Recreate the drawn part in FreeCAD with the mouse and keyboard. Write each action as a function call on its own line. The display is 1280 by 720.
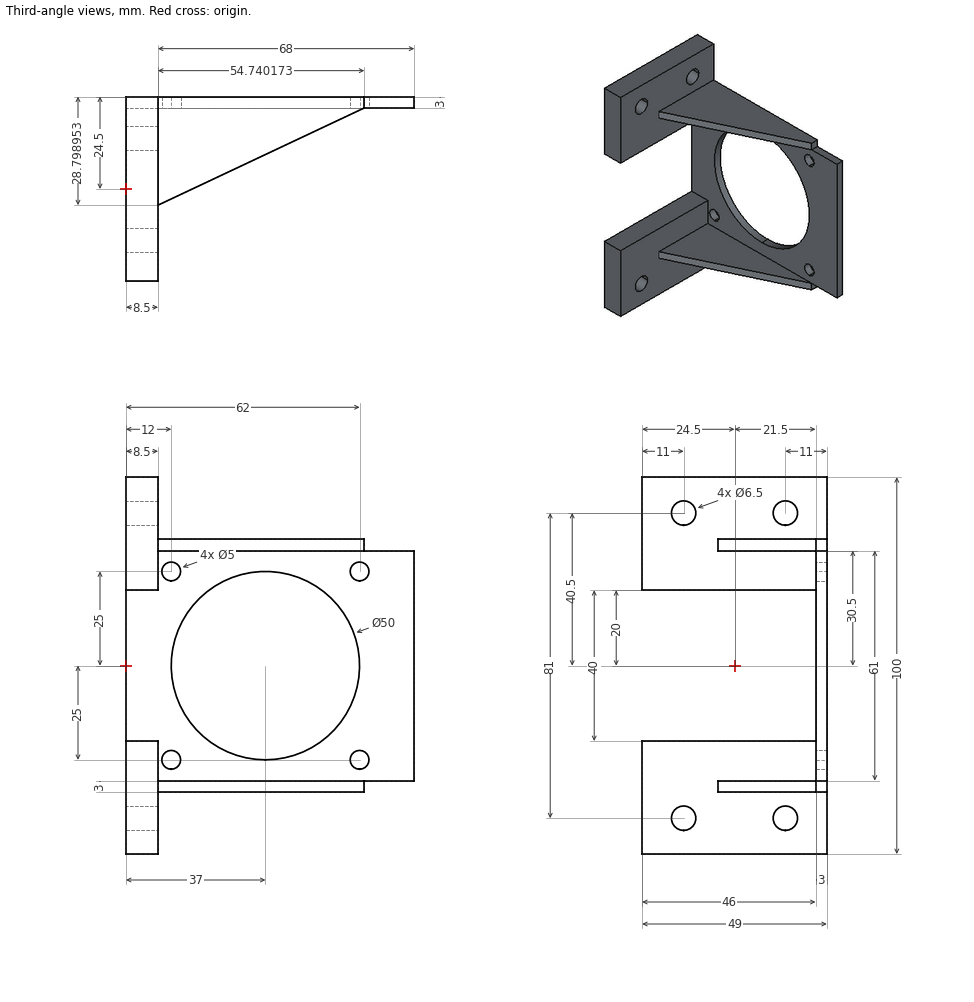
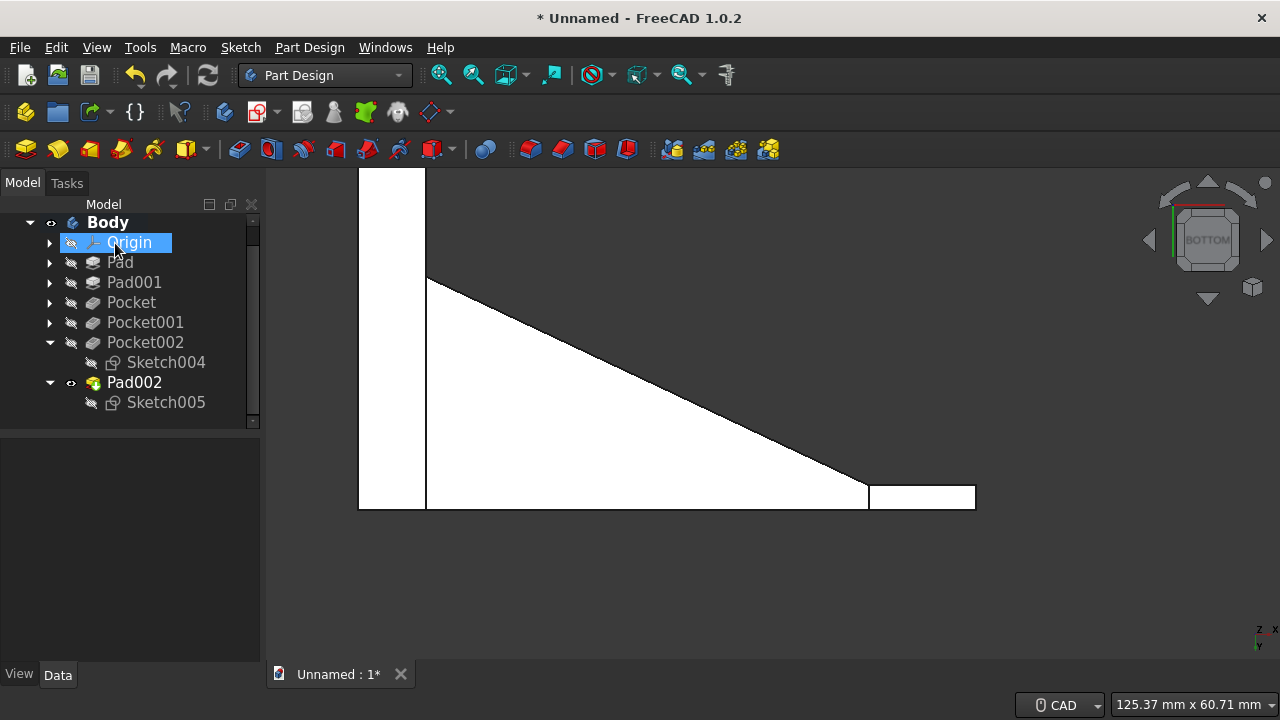
click(442, 76)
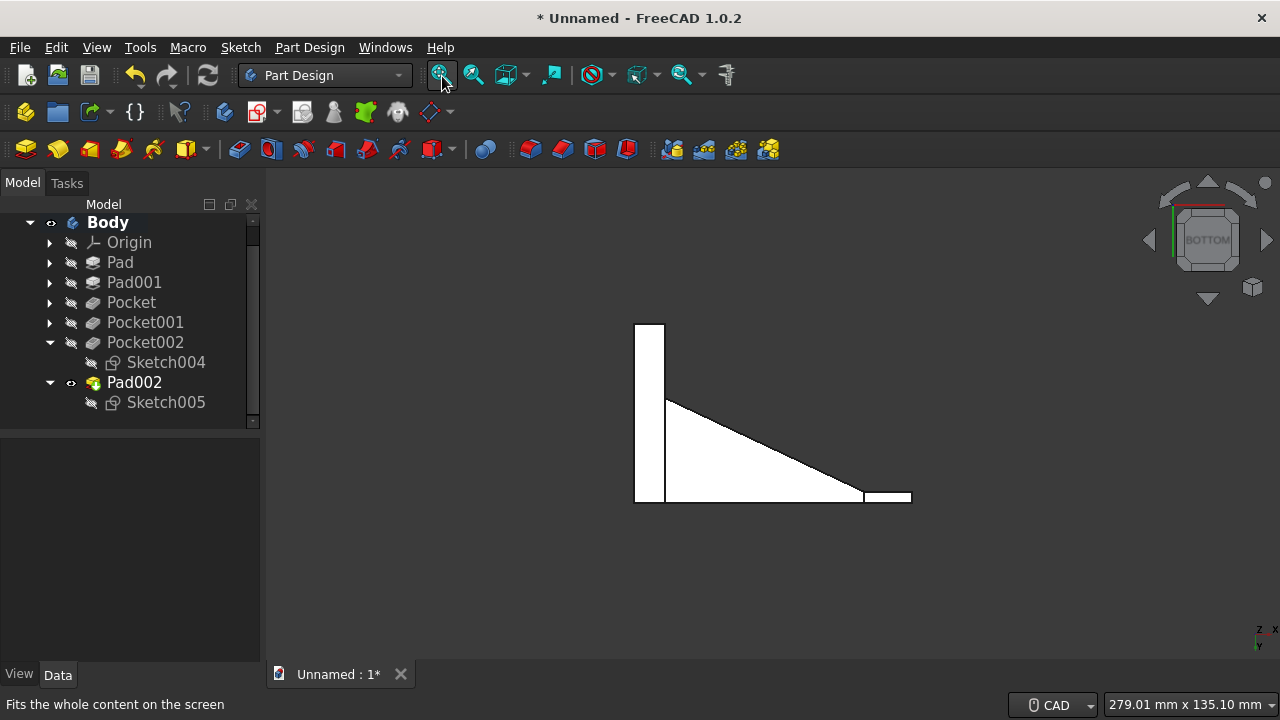
click(116, 383)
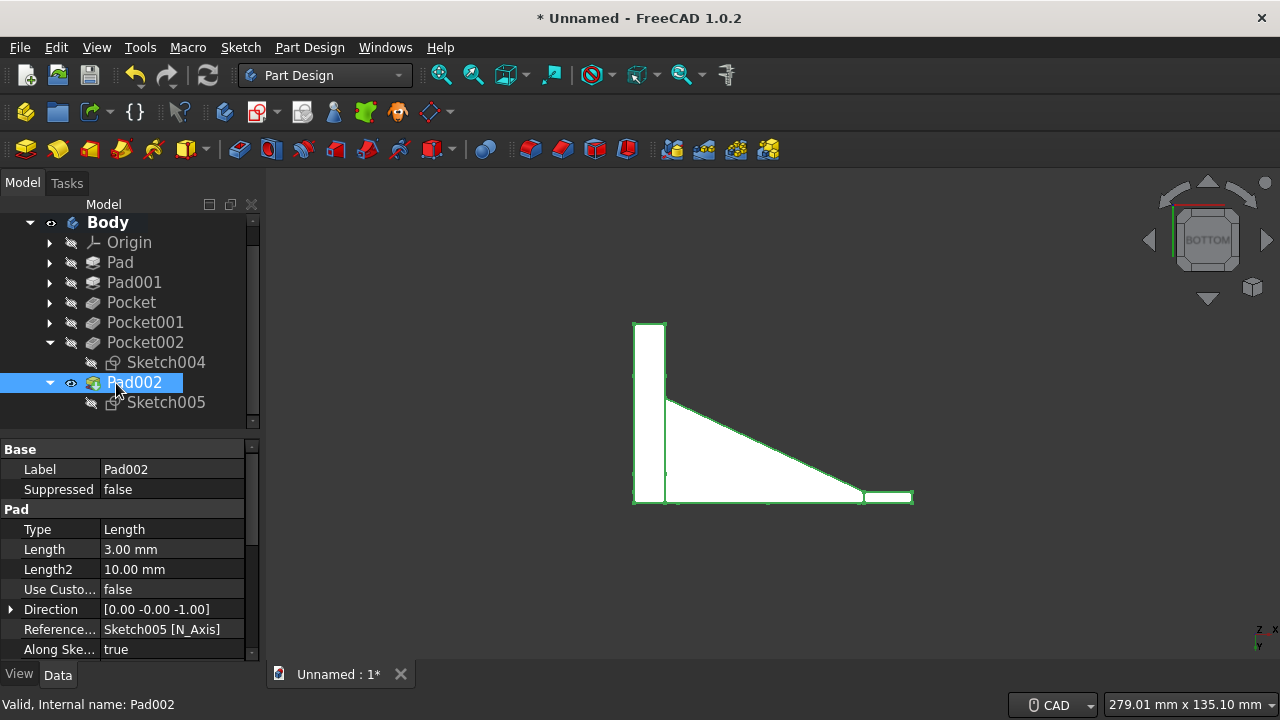
click(672, 150)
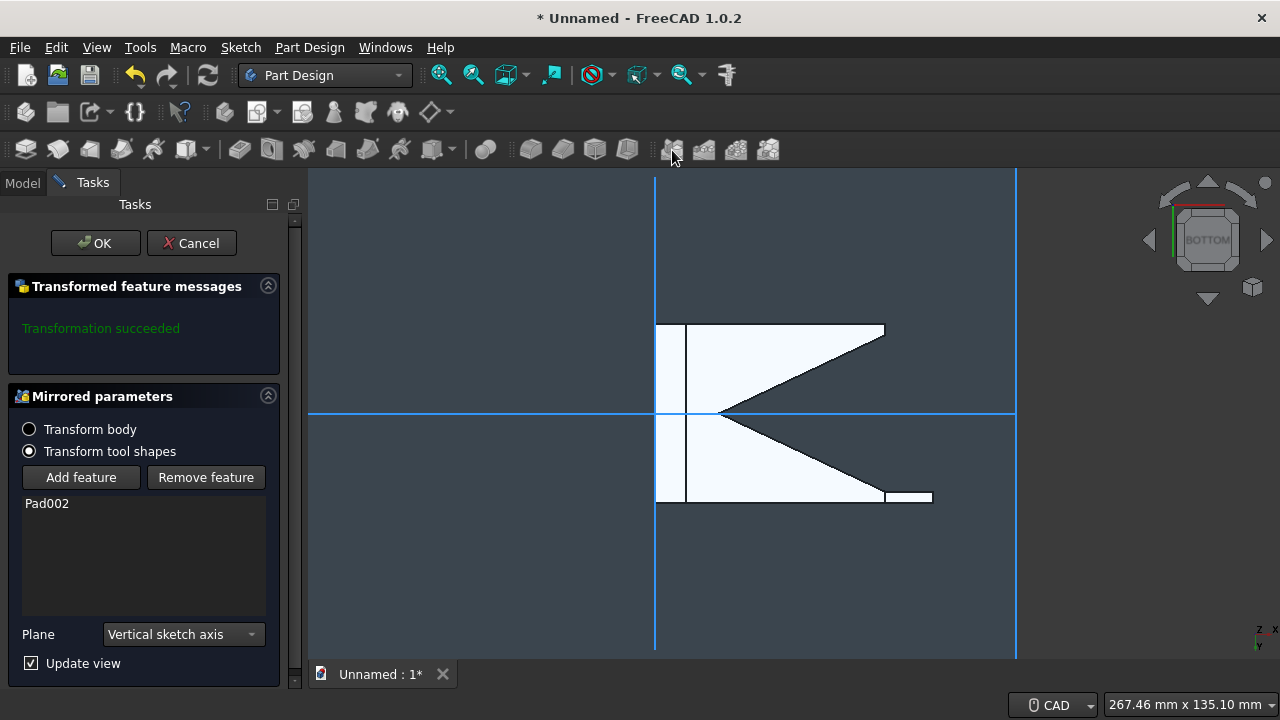
click(184, 634)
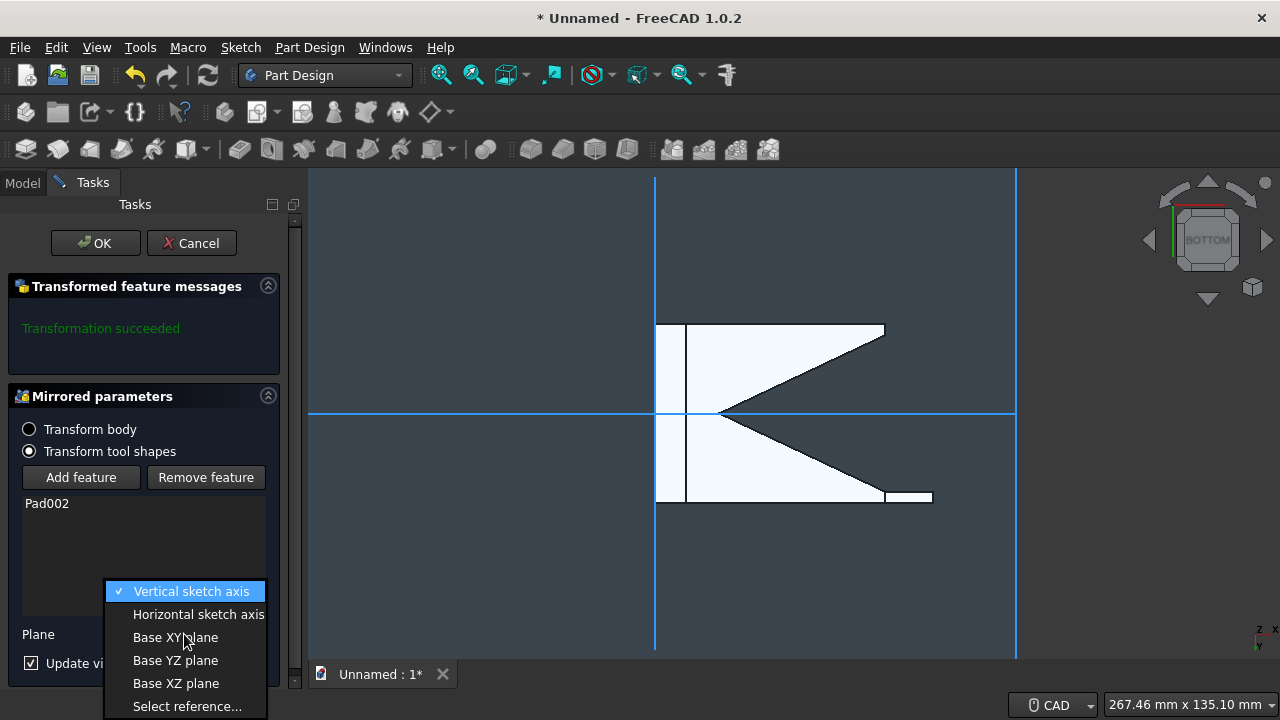
click(184, 638)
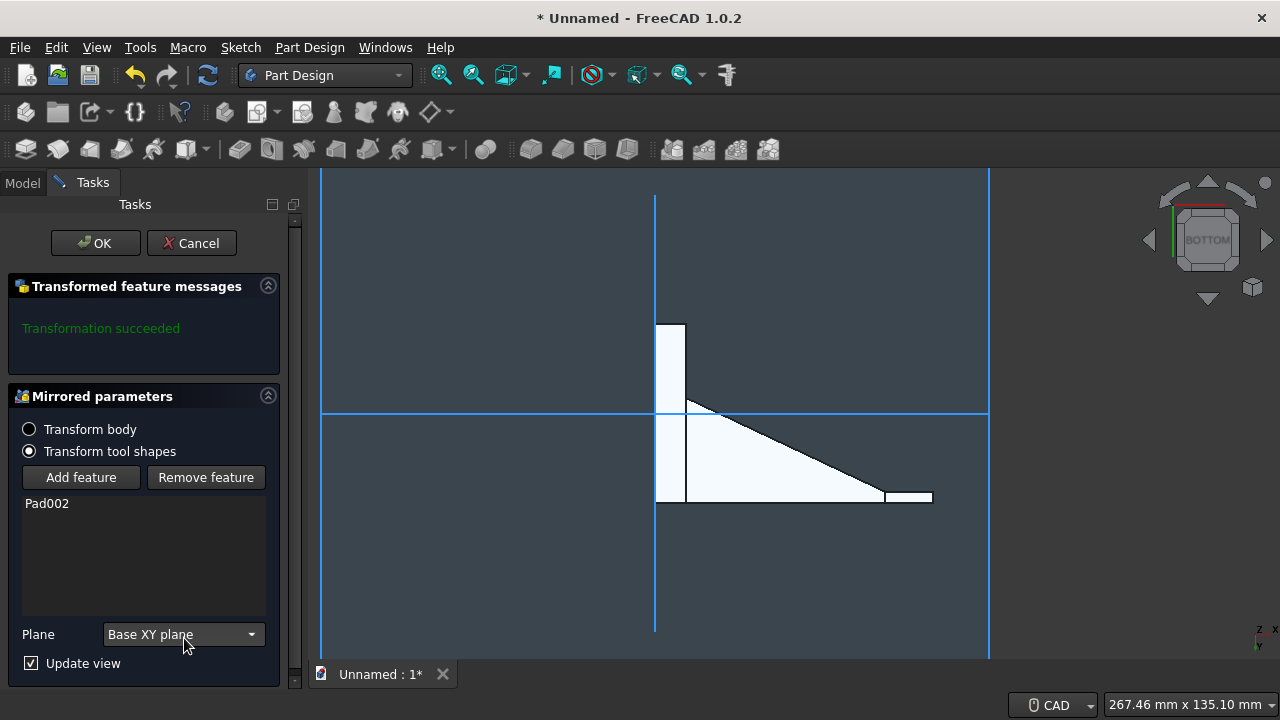
click(96, 243)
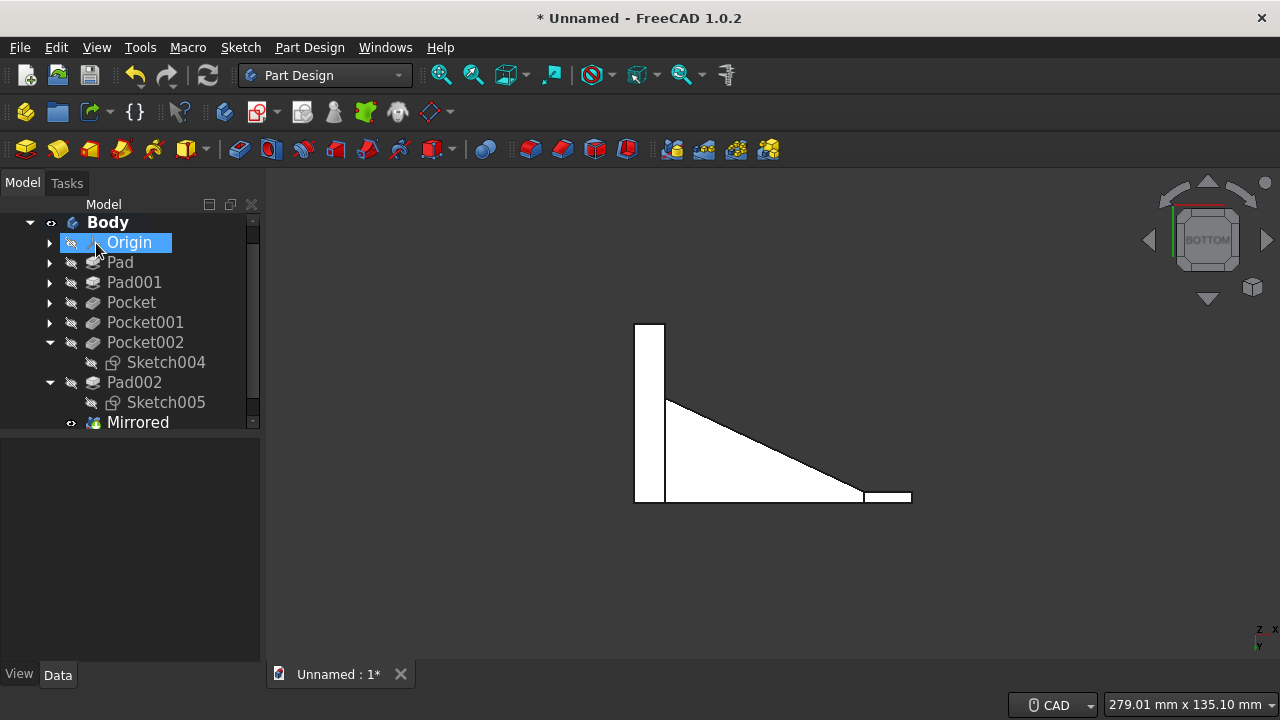
key(0)